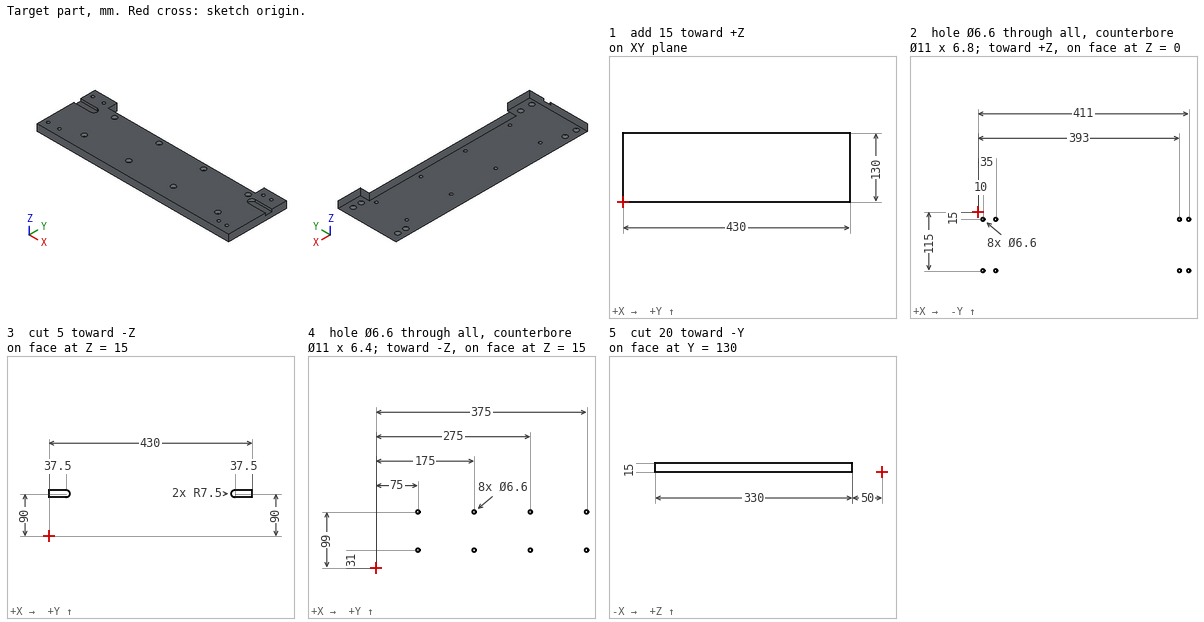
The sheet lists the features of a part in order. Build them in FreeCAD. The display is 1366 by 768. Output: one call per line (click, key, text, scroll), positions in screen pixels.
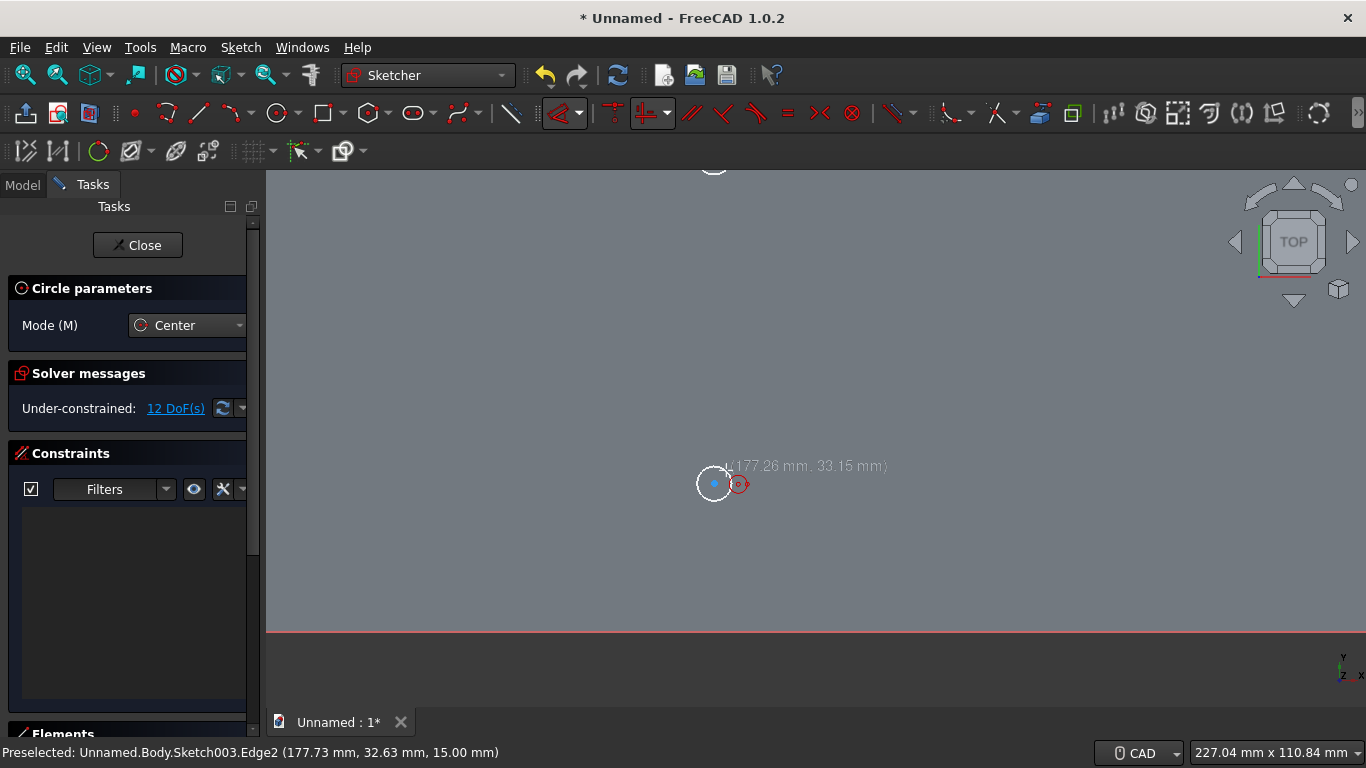
scroll(726, 470, down, 5)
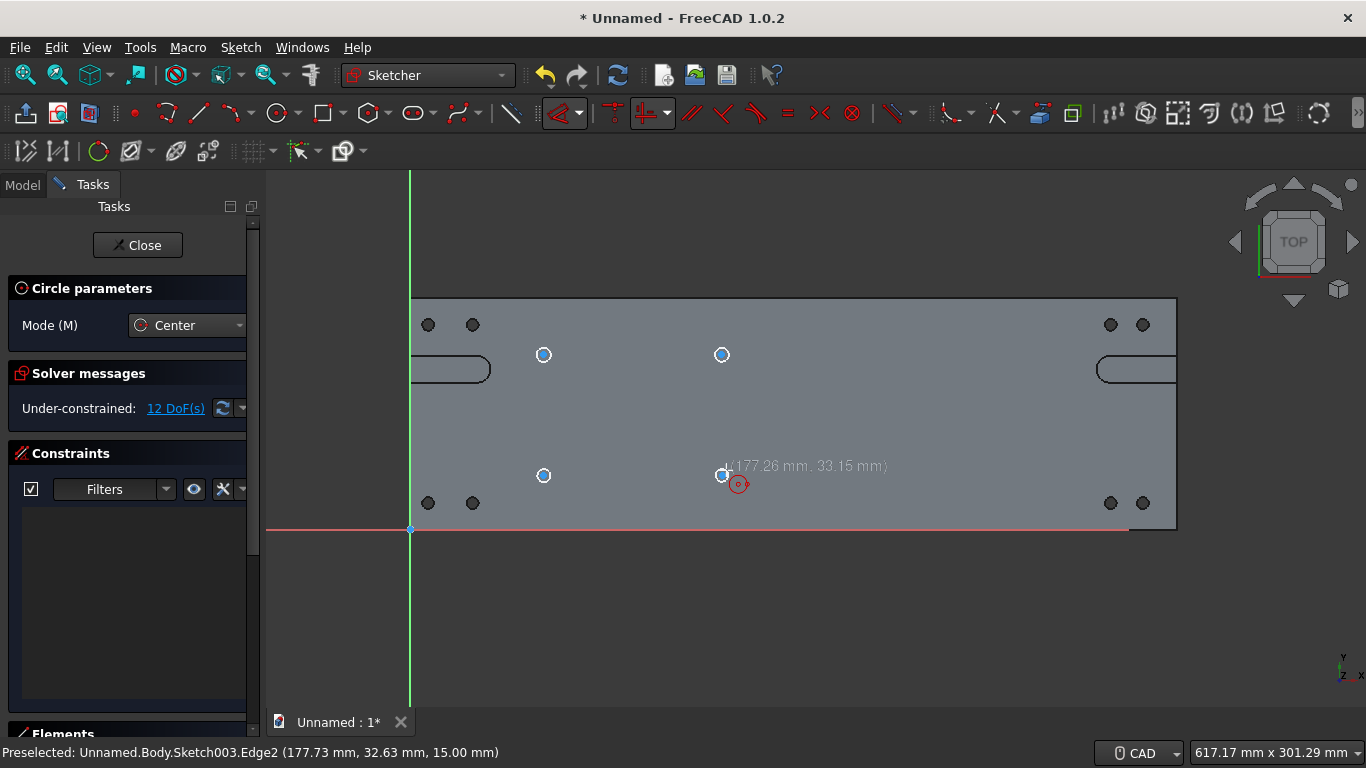
scroll(900, 353, up, 7)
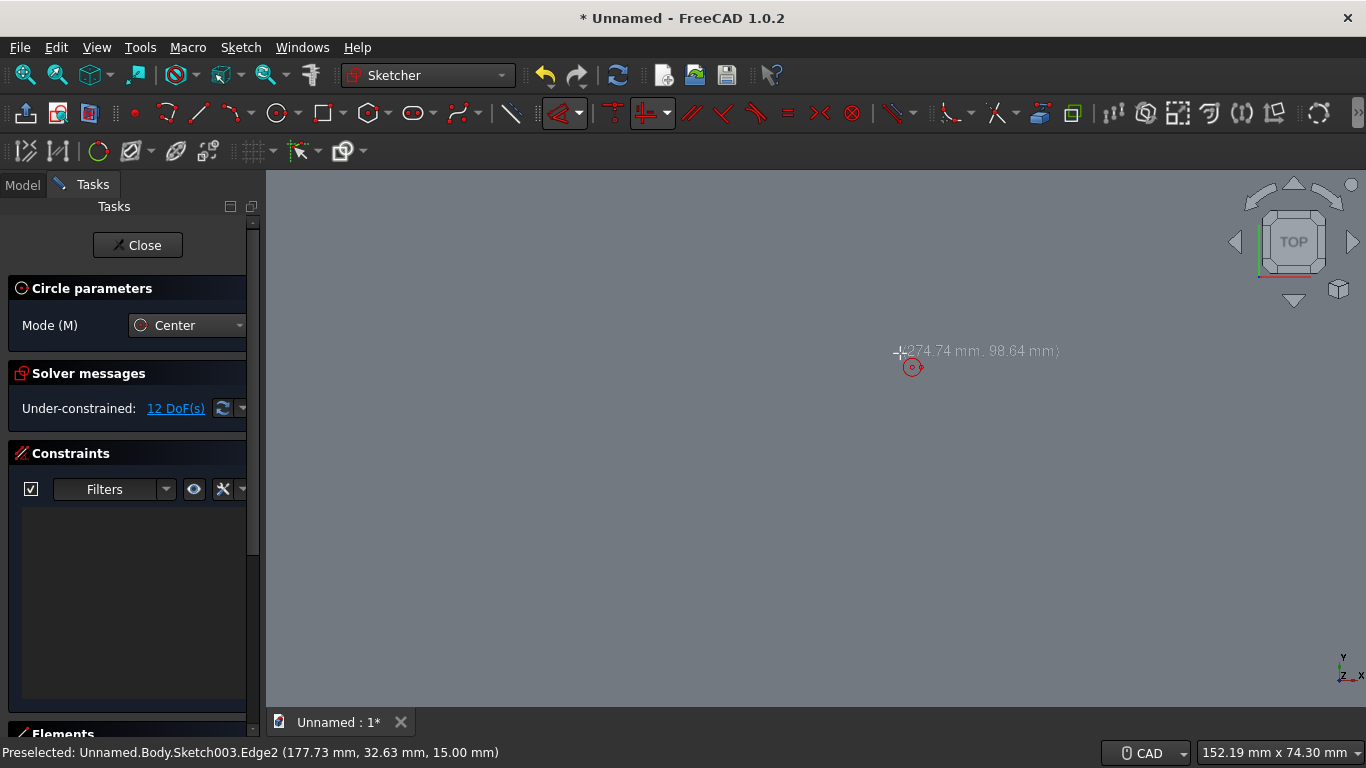
scroll(901, 353, down, 7)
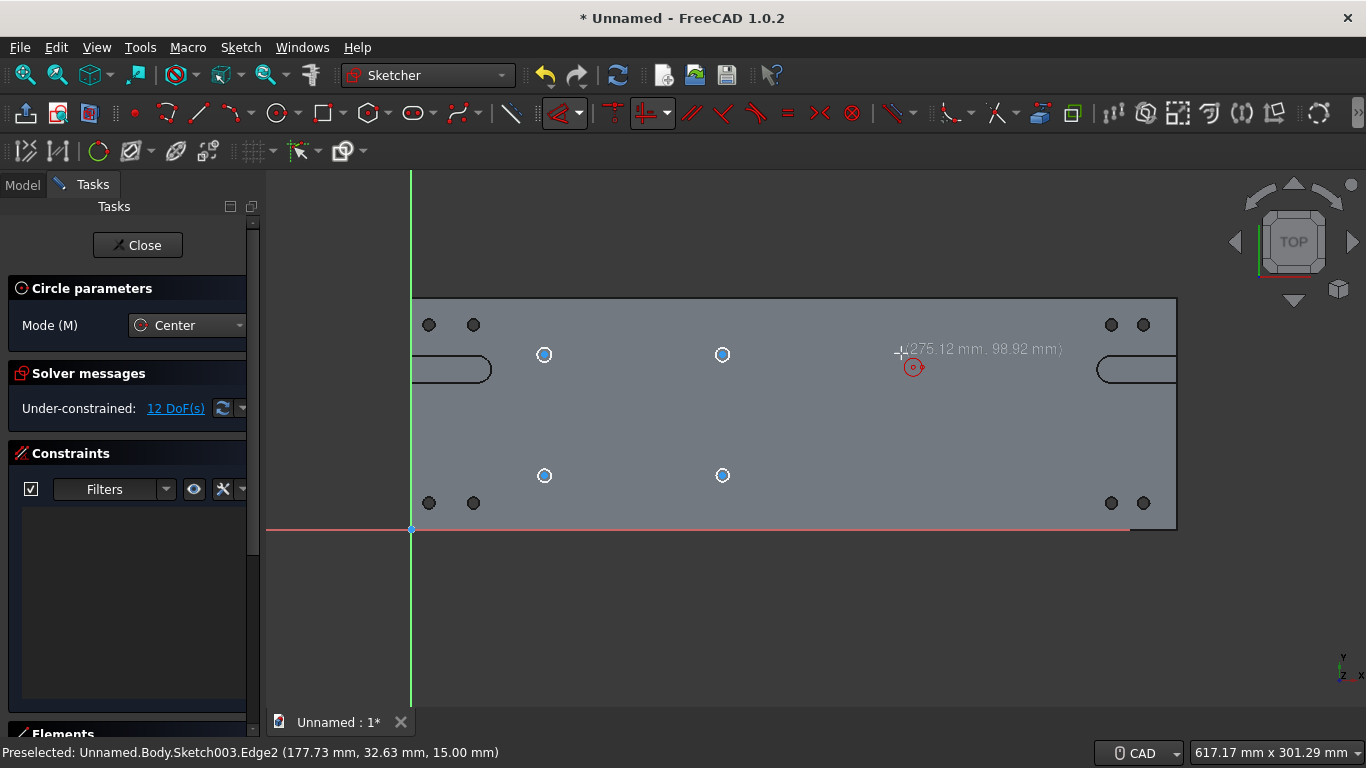
click(901, 353)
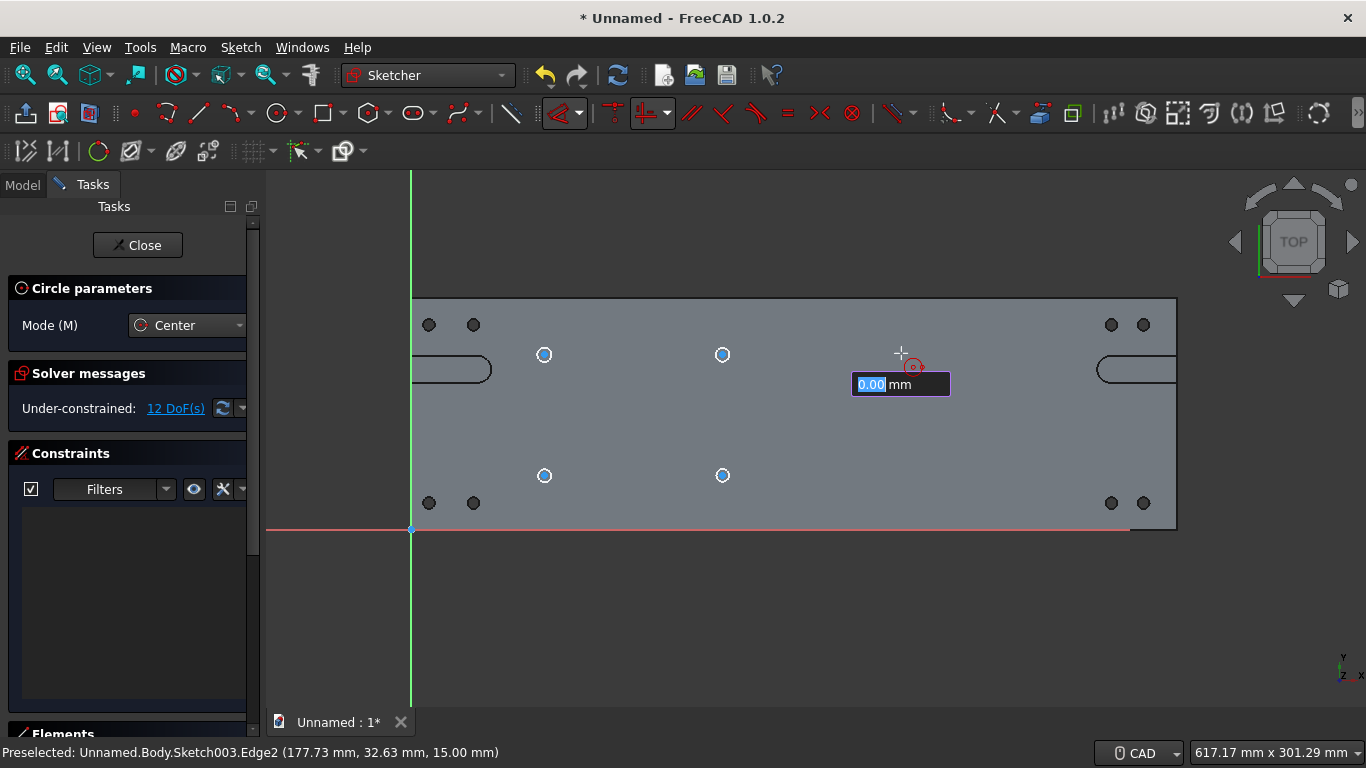
scroll(905, 349, up, 5)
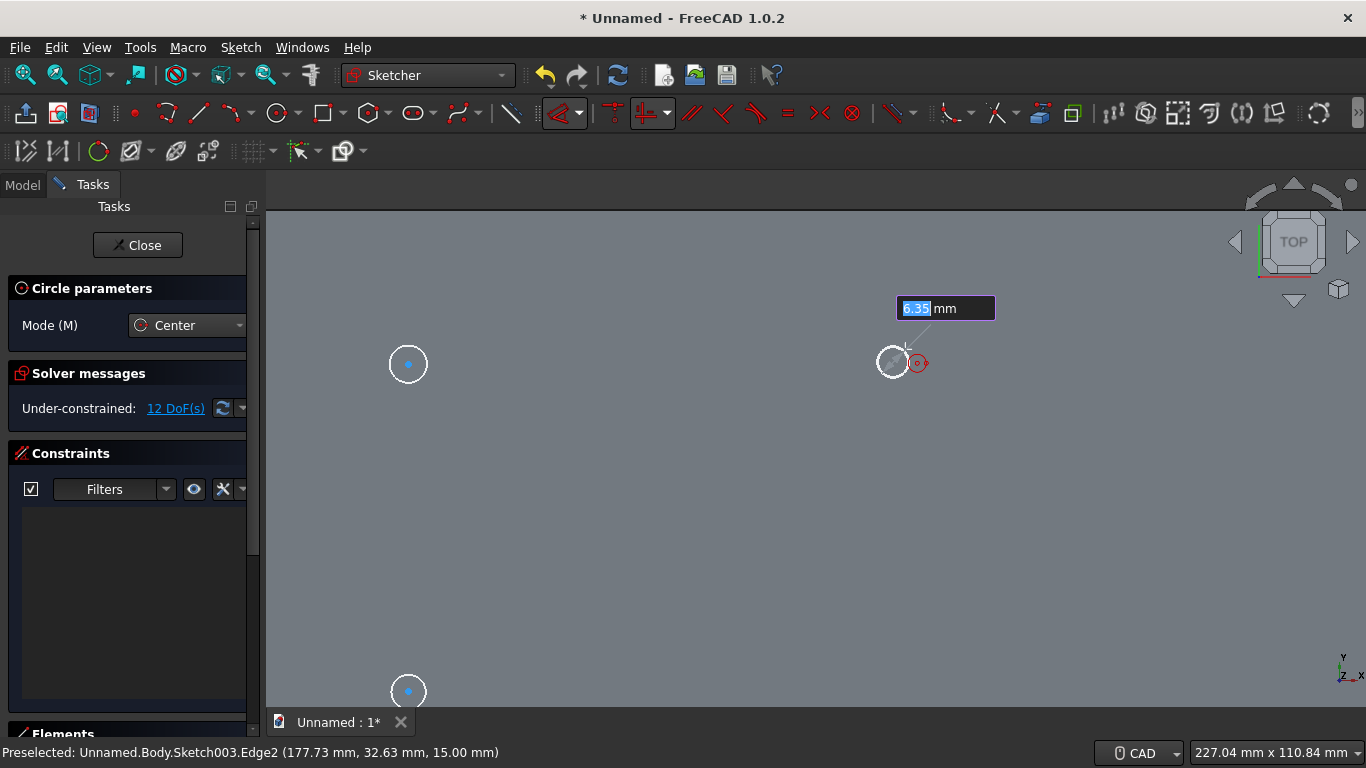
click(905, 349)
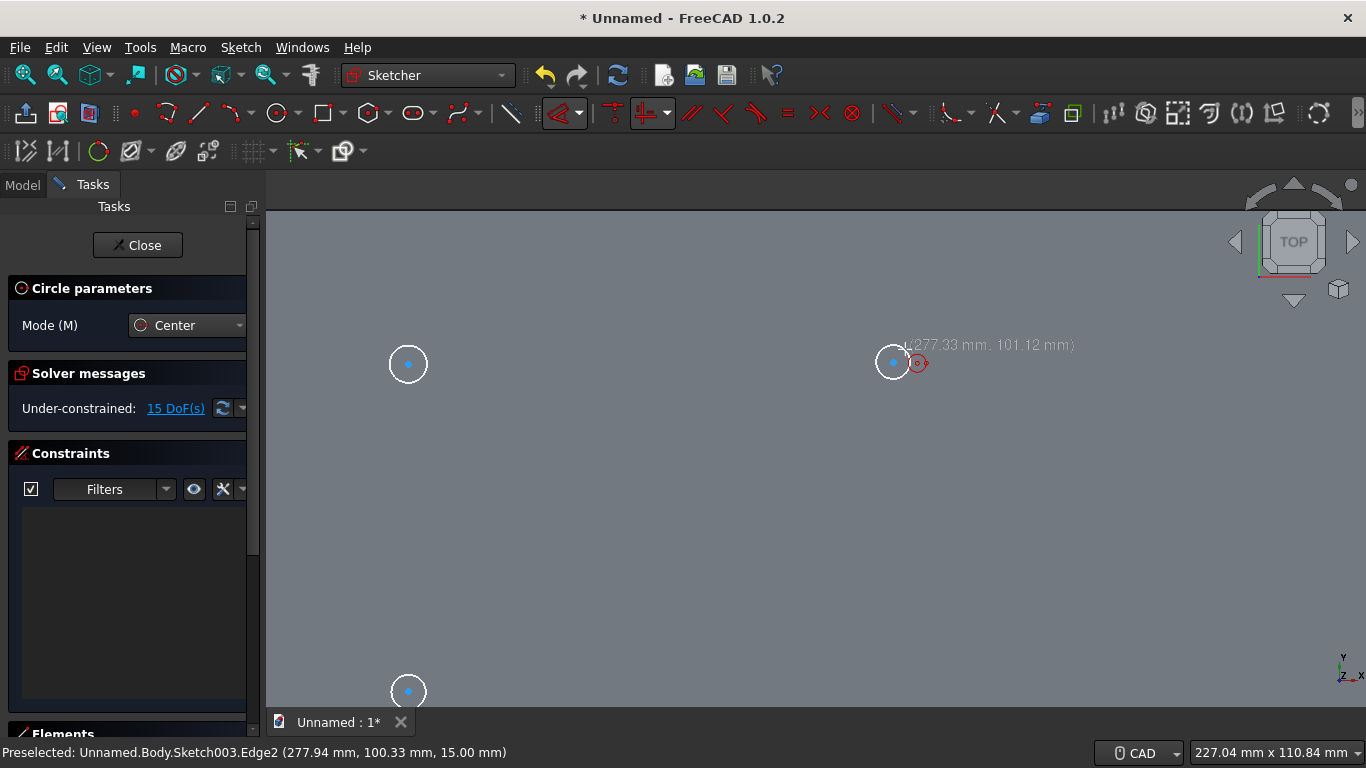
scroll(904, 349, down, 5)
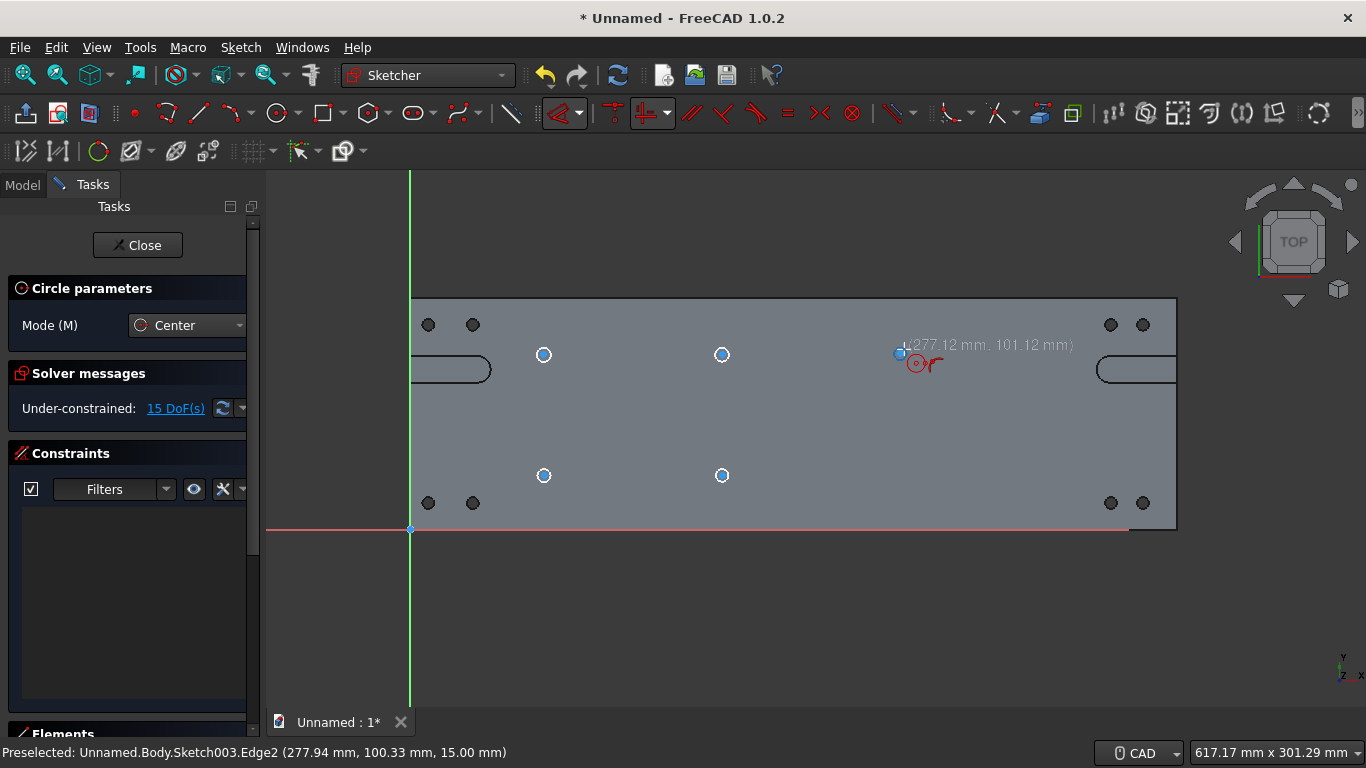
scroll(901, 475, up, 7)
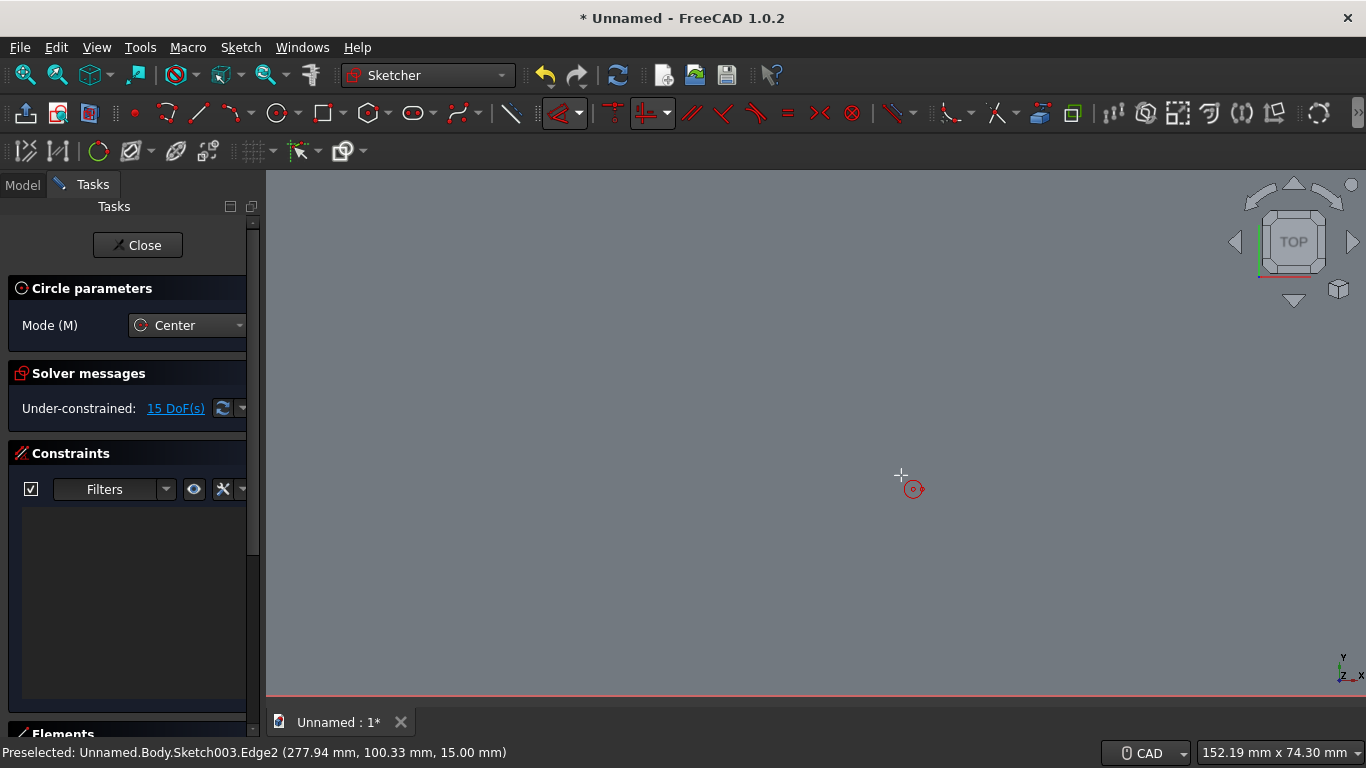
scroll(901, 475, down, 7)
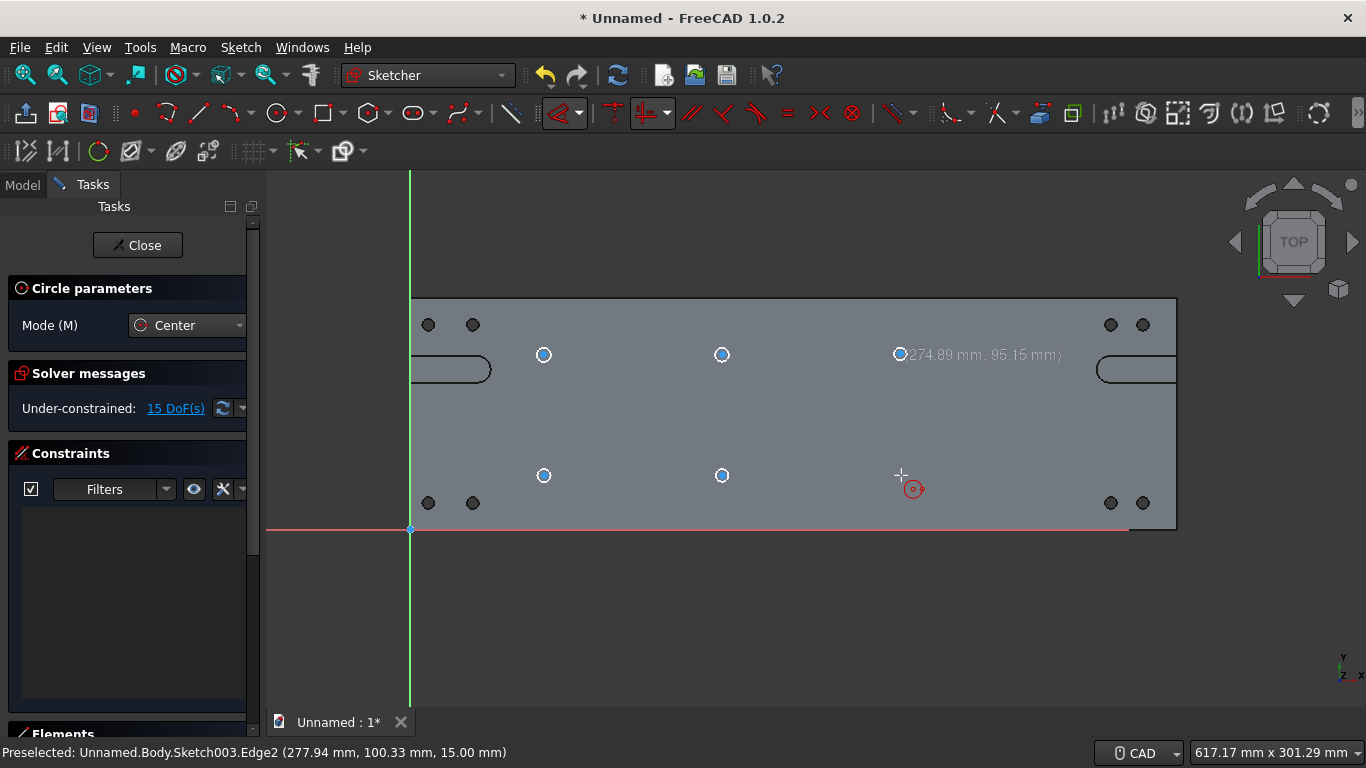
click(901, 475)